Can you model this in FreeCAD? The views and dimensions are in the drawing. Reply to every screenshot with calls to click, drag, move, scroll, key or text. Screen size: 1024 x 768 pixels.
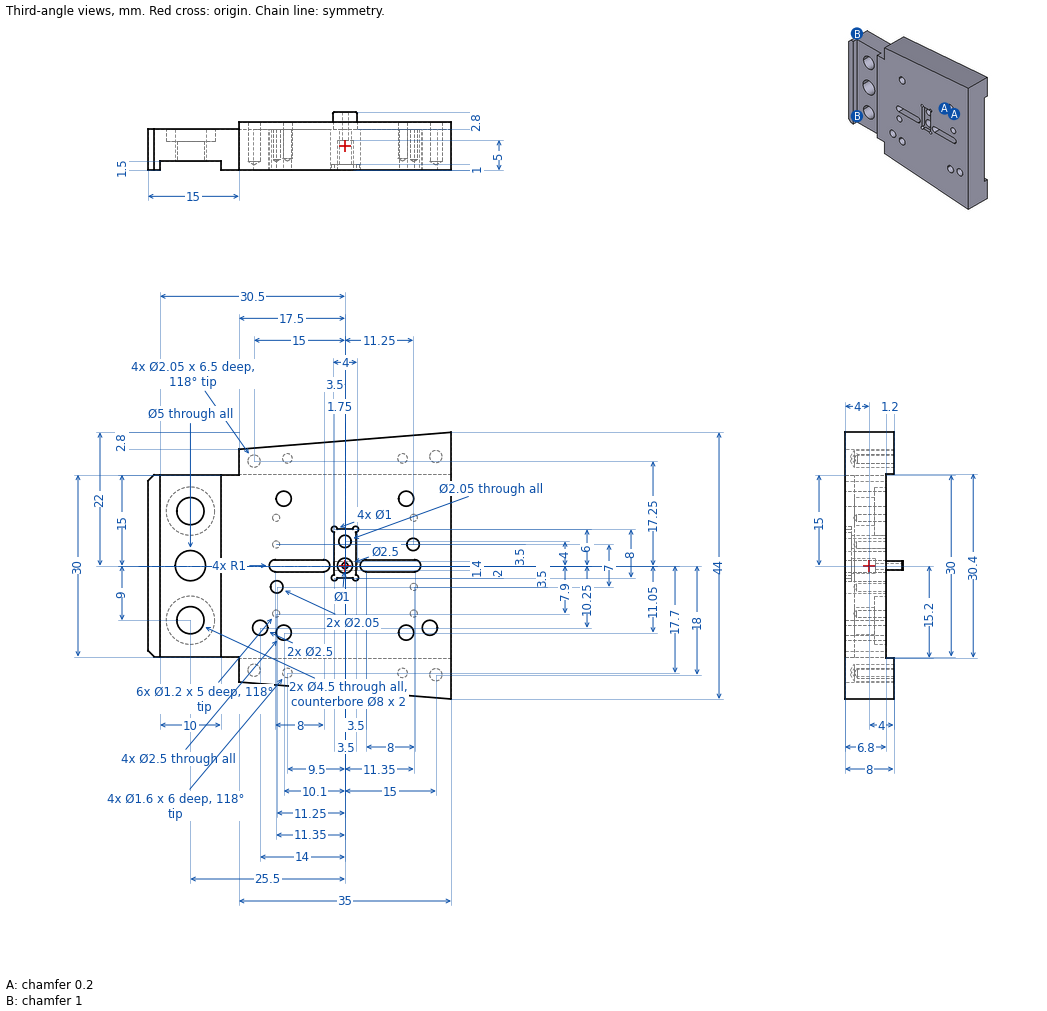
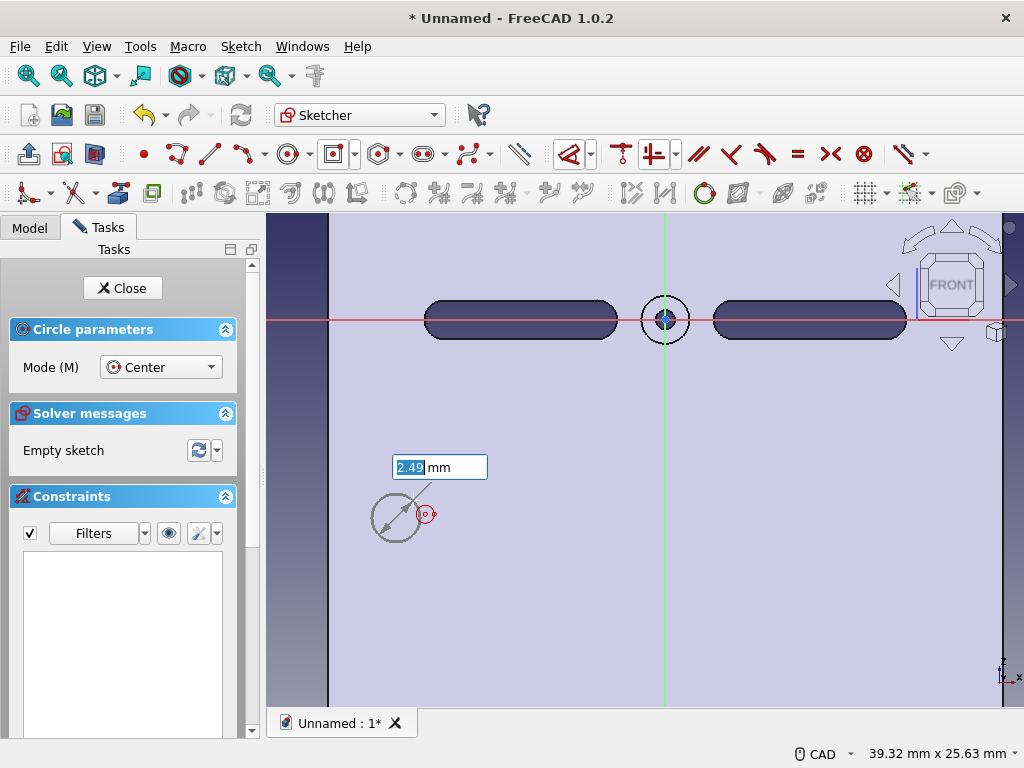
text(2.5)
key(Return)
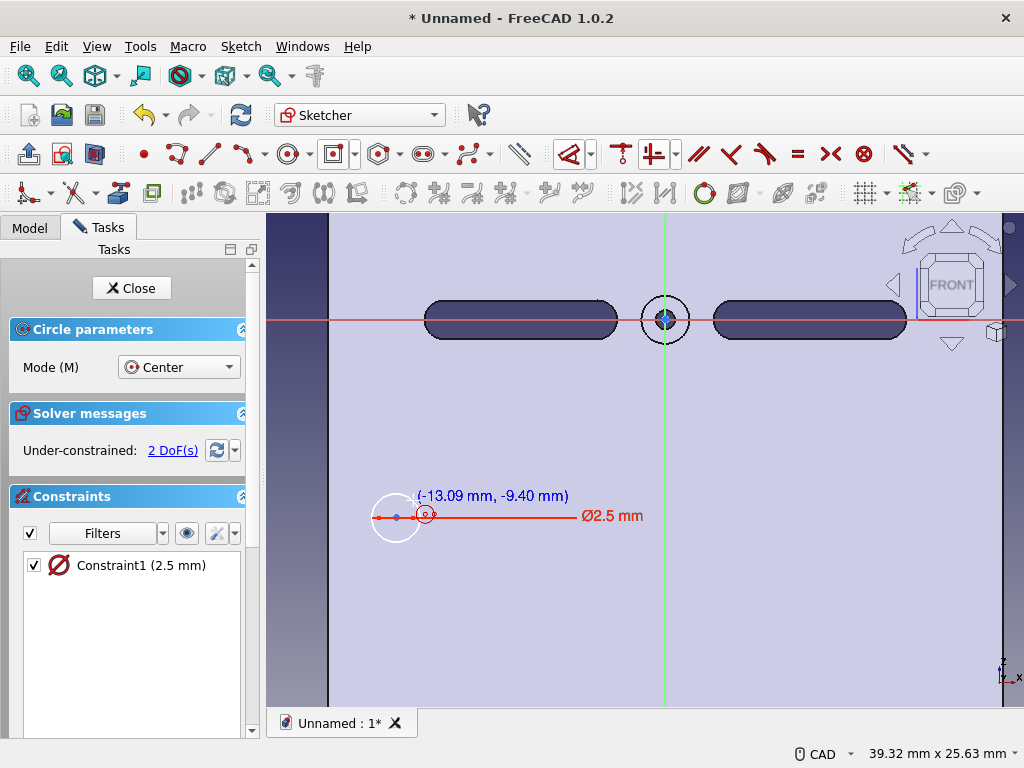
scroll(396, 520, down, 2)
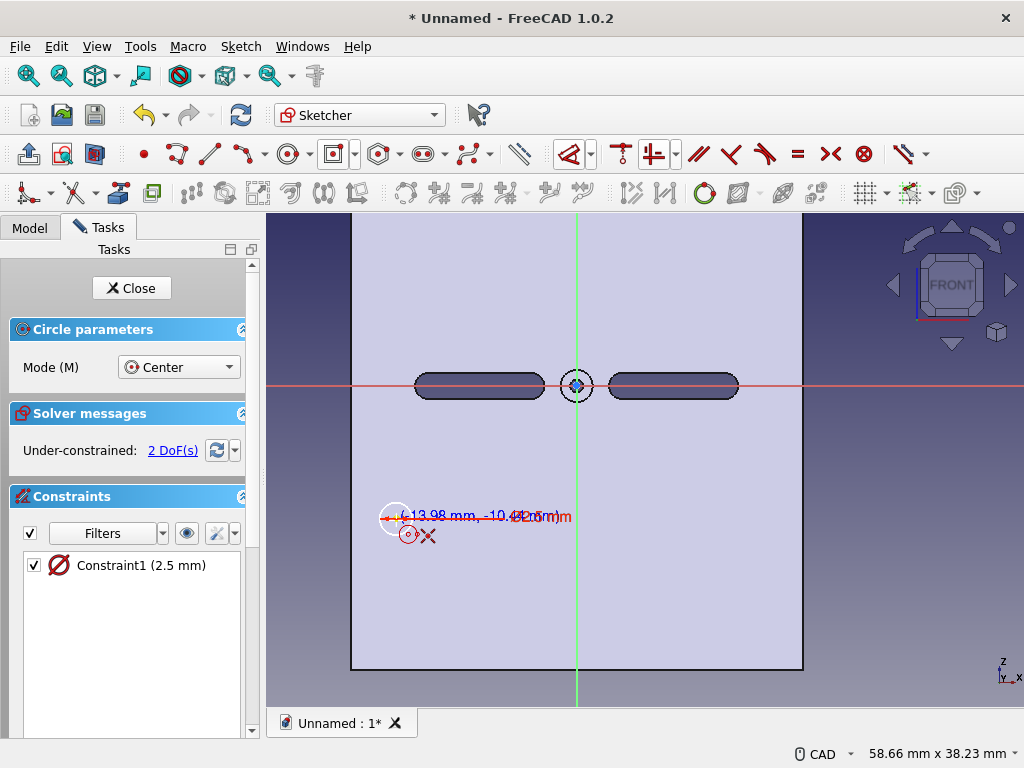
scroll(758, 518, up, 2)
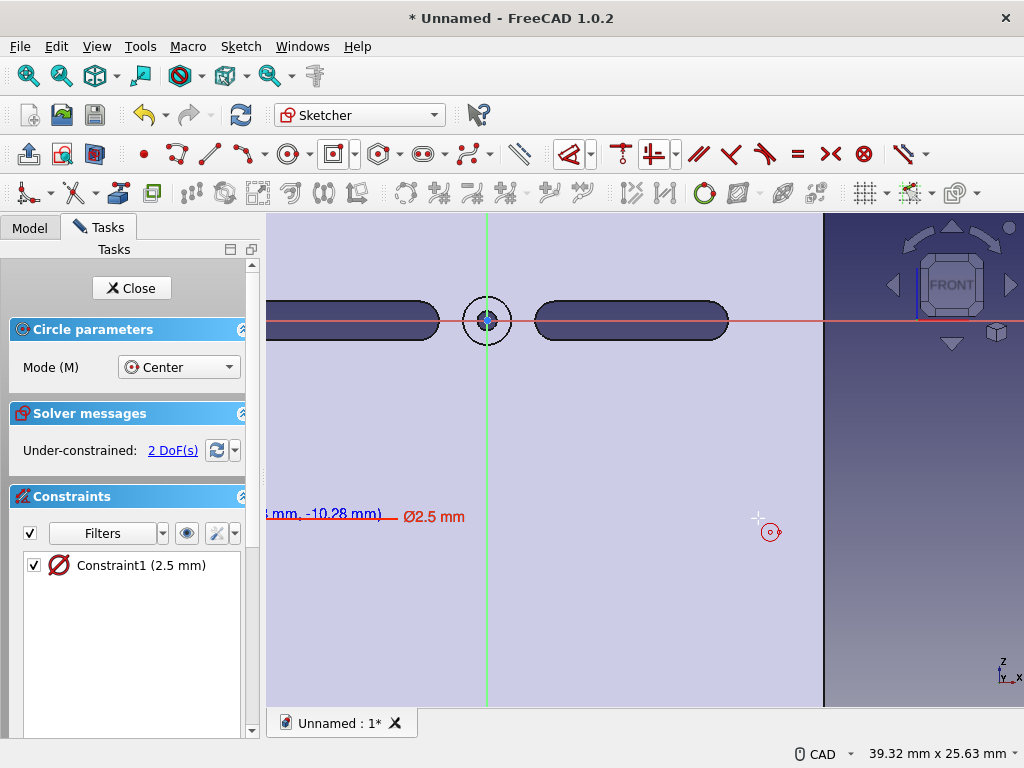
click(757, 518)
move(774, 501)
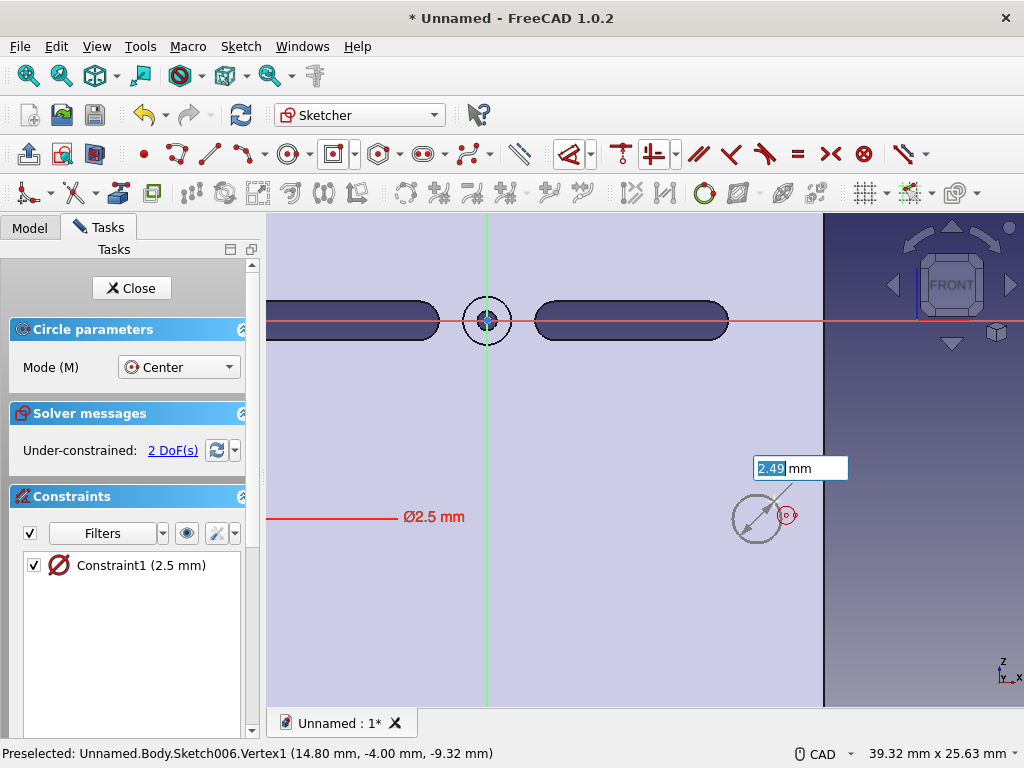
text(2.5)
key(Return)
key(Escape)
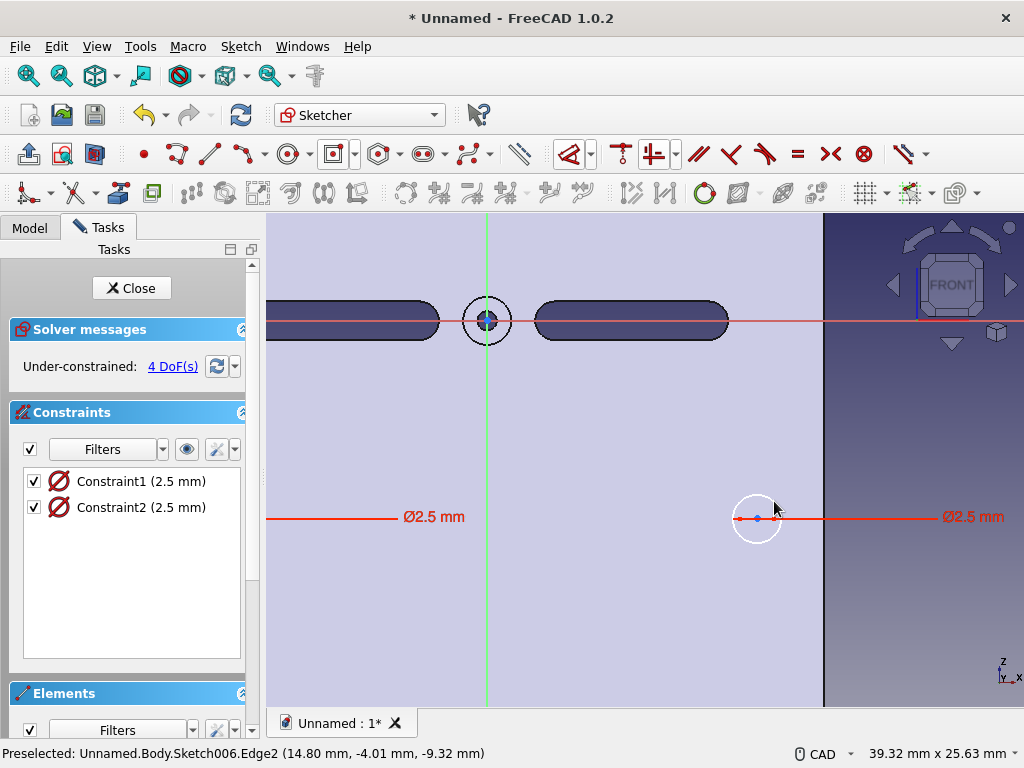
scroll(758, 518, down, 2)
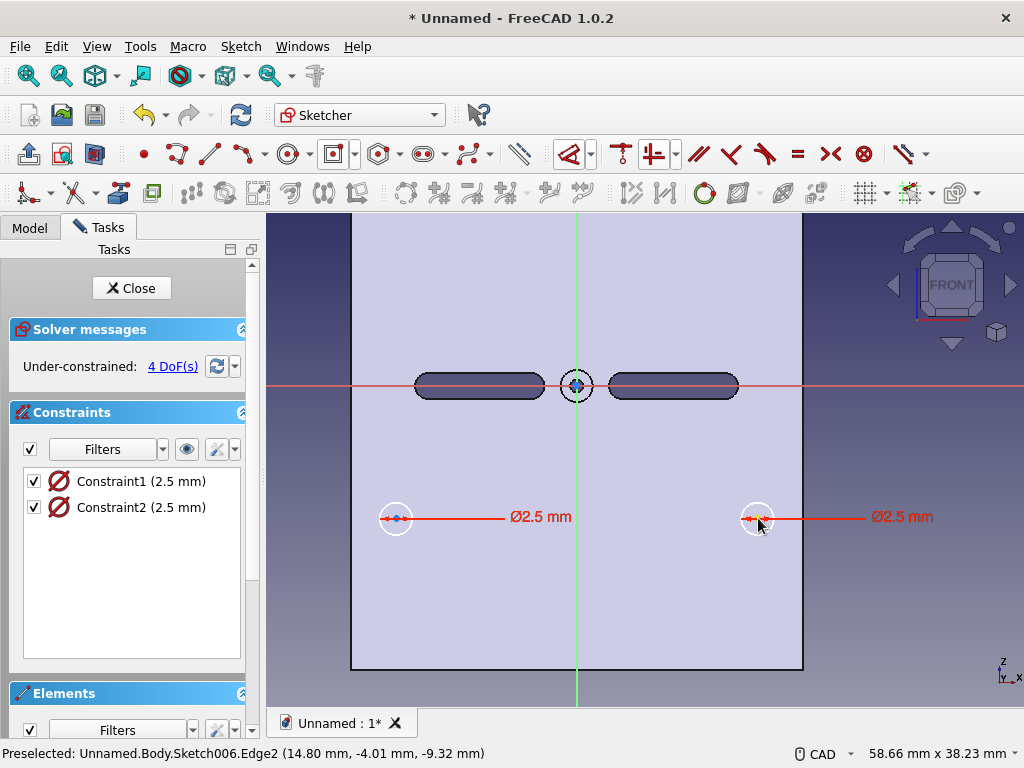
click(396, 519)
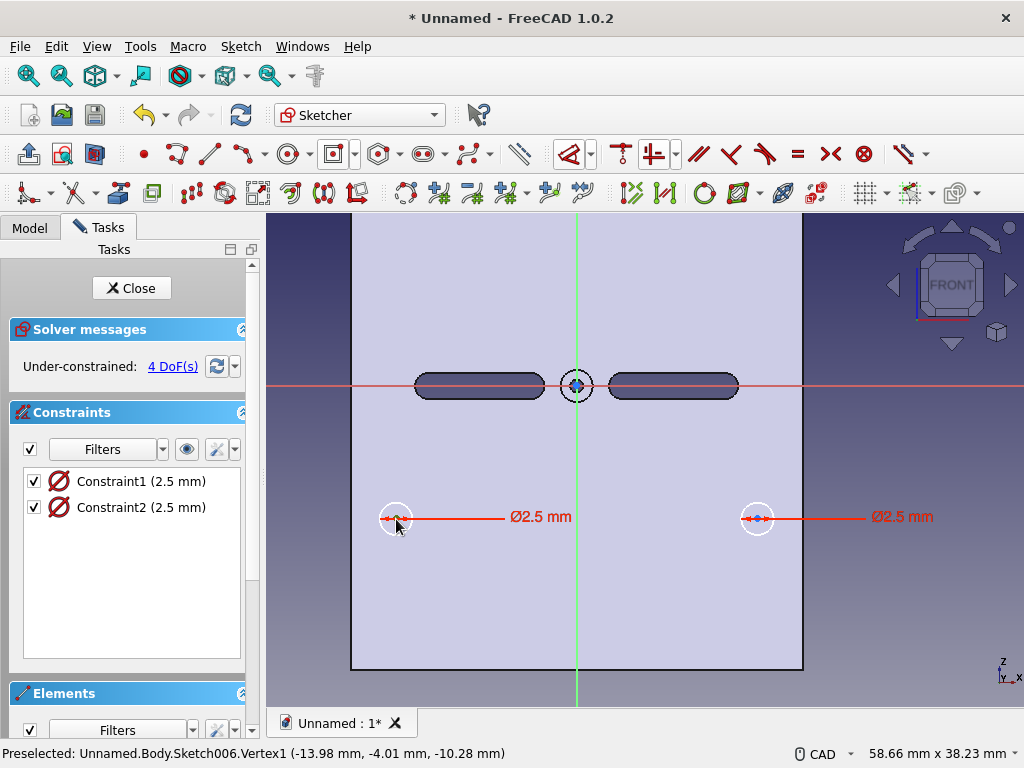
click(758, 519)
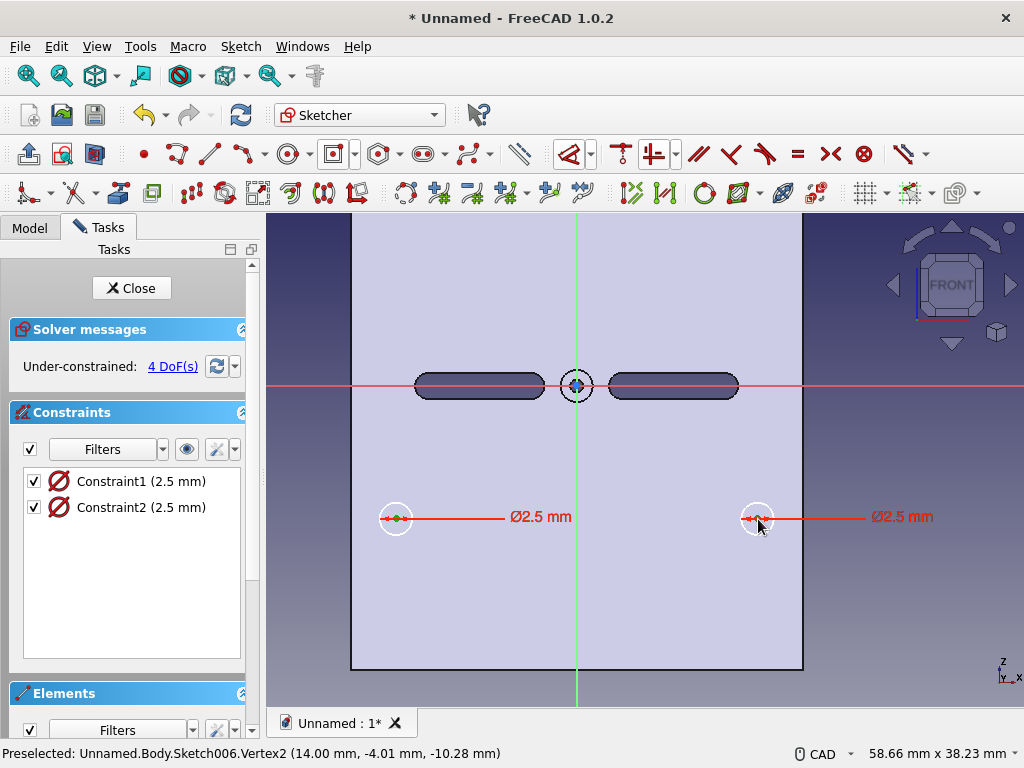
click(577, 648)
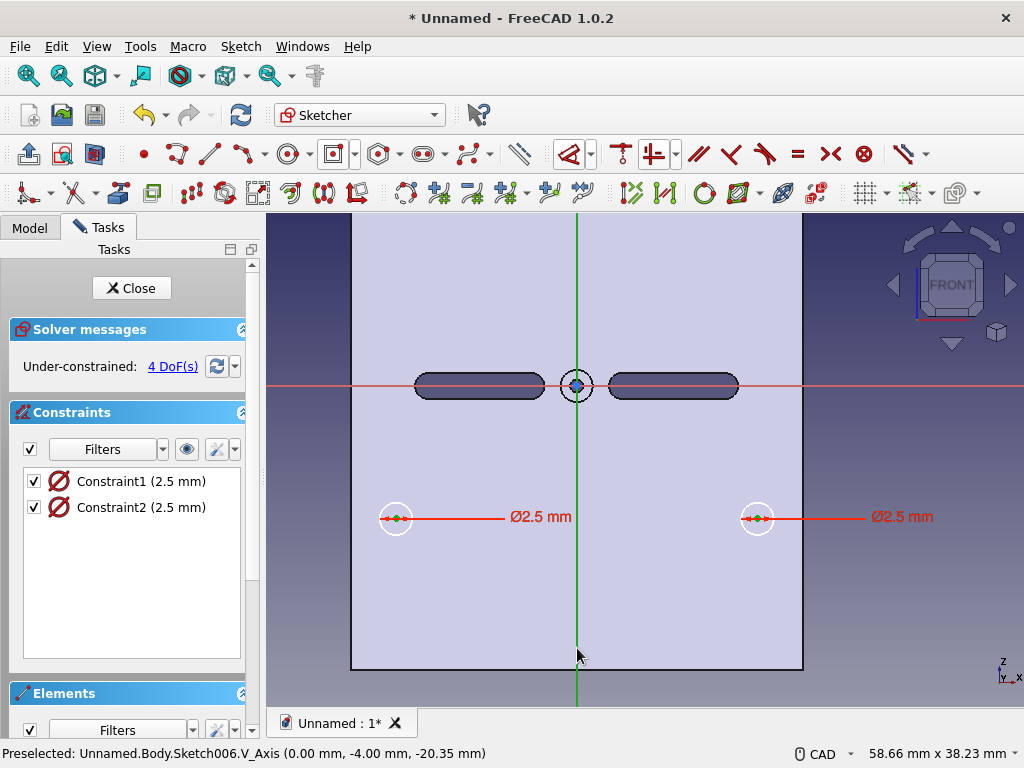
click(831, 154)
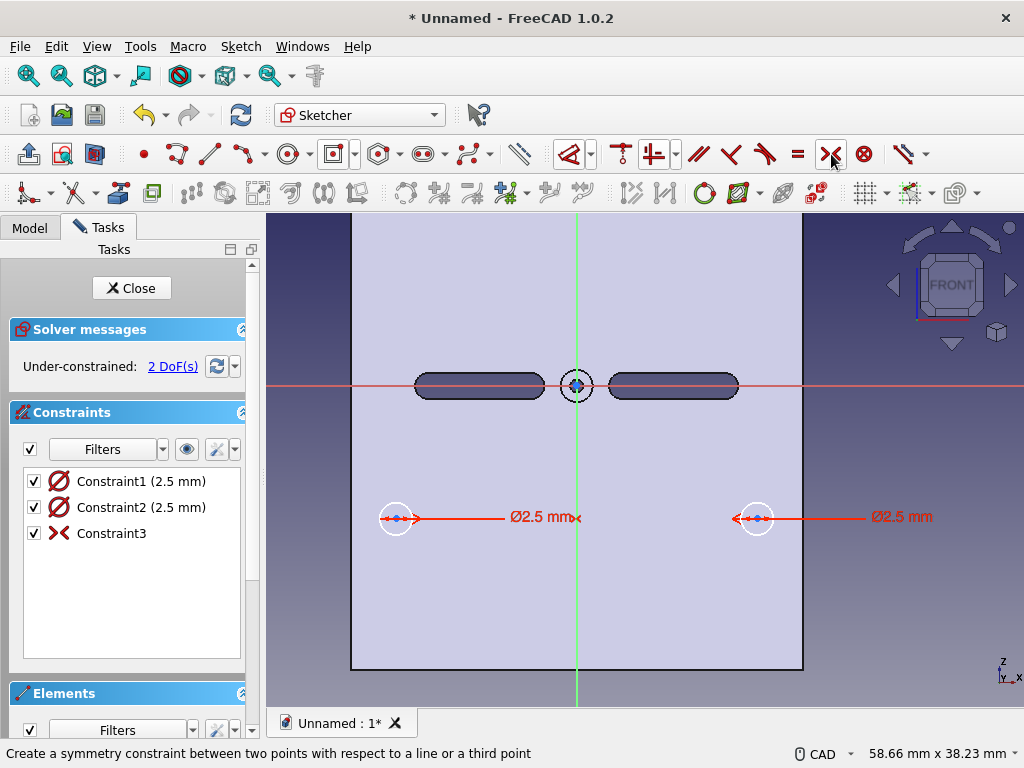
click(396, 519)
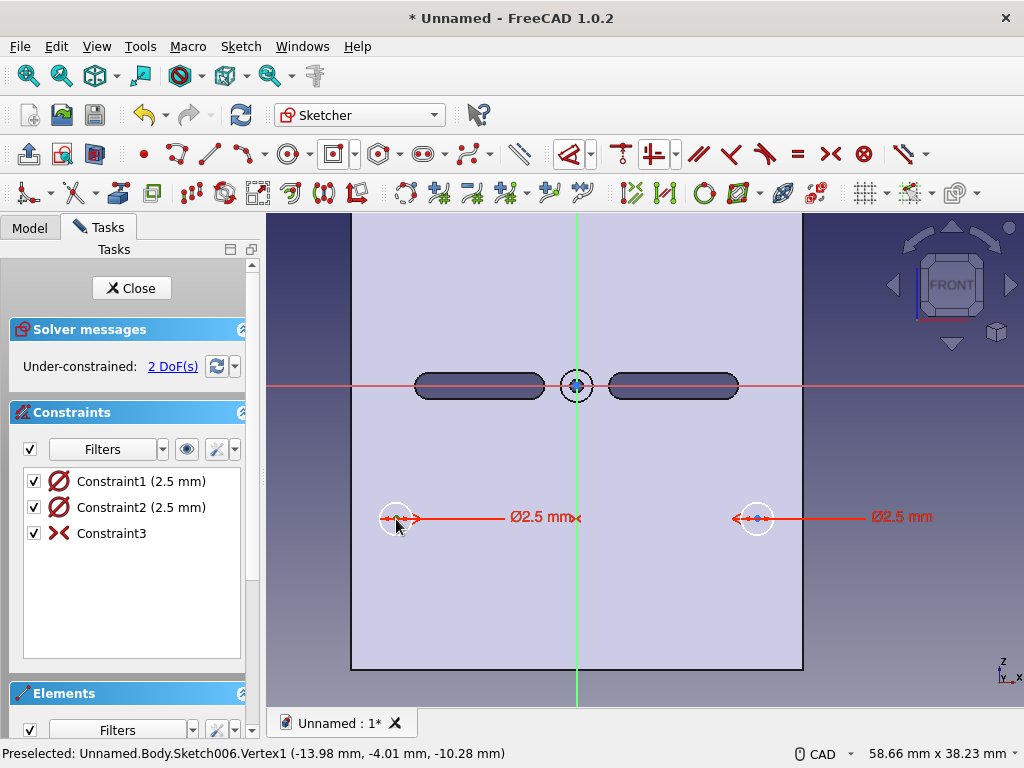
click(590, 154)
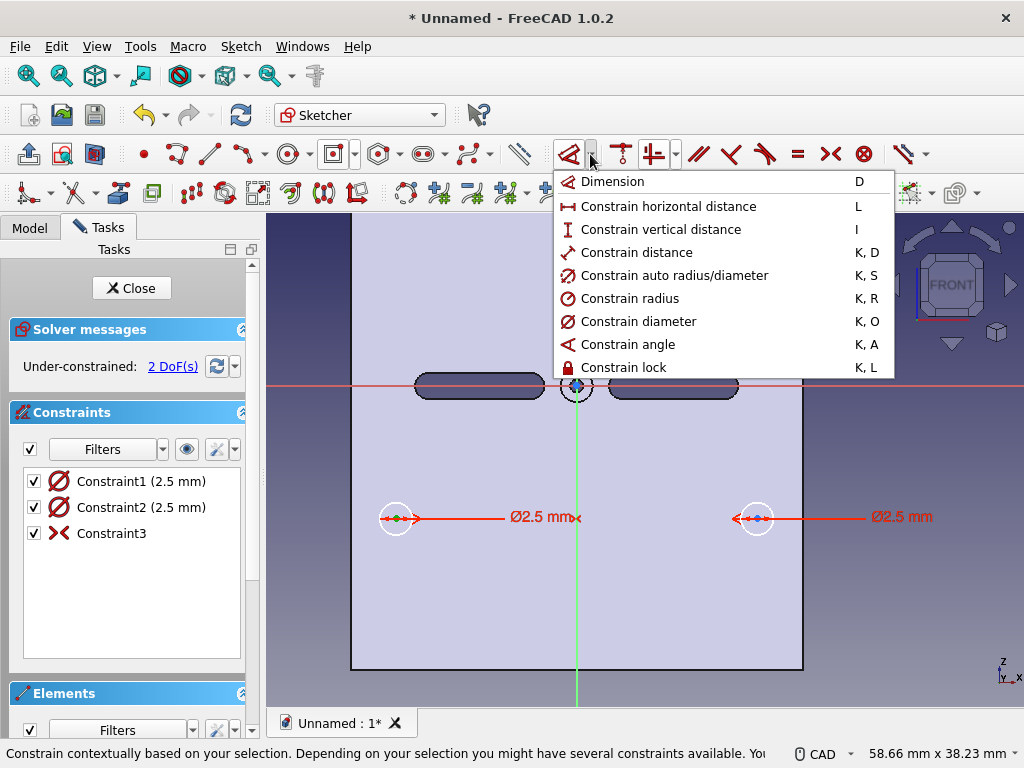
click(724, 206)